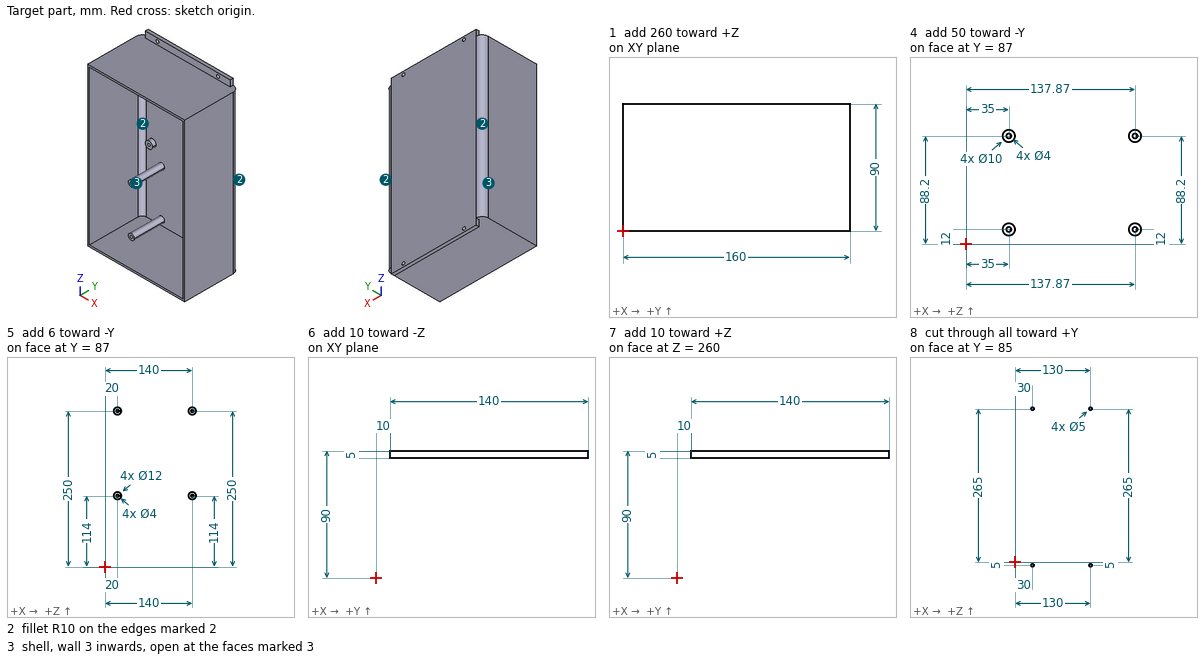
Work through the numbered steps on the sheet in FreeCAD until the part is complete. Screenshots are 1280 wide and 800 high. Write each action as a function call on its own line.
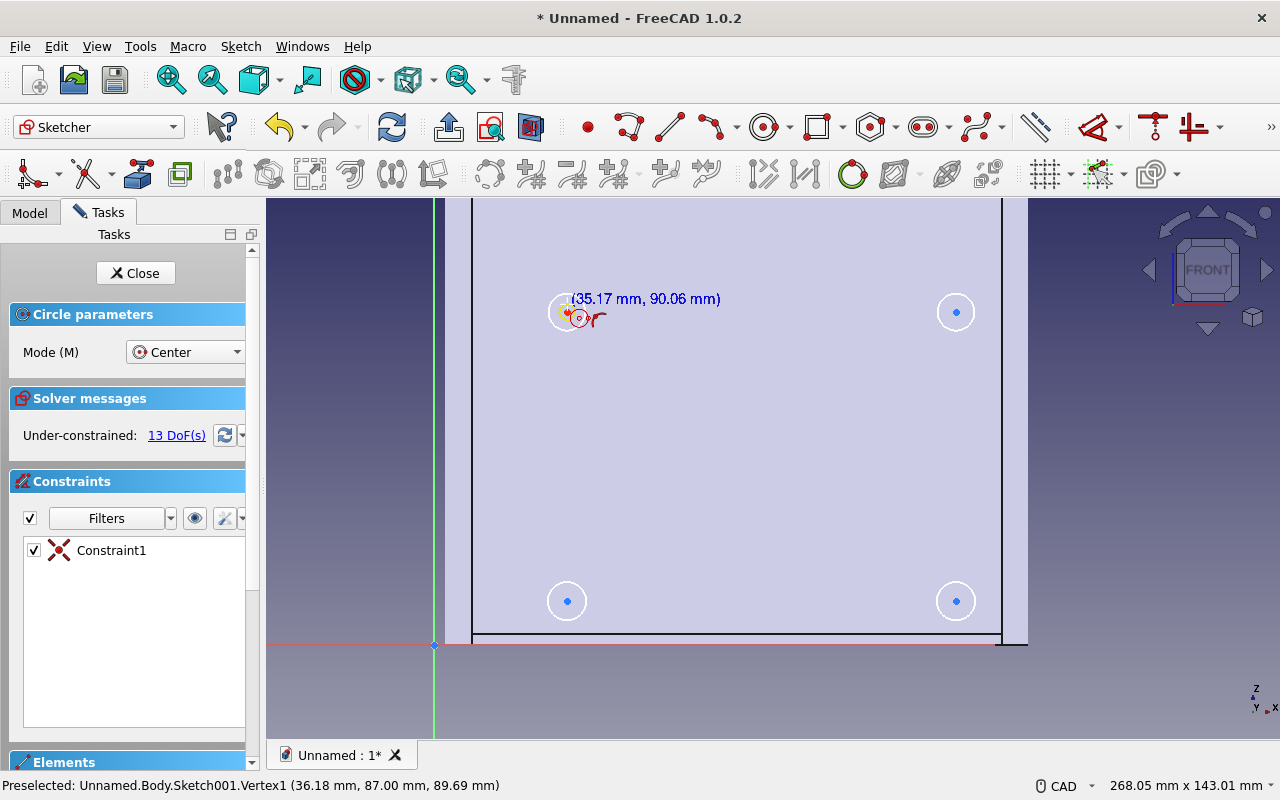
scroll(567, 600, up, 6)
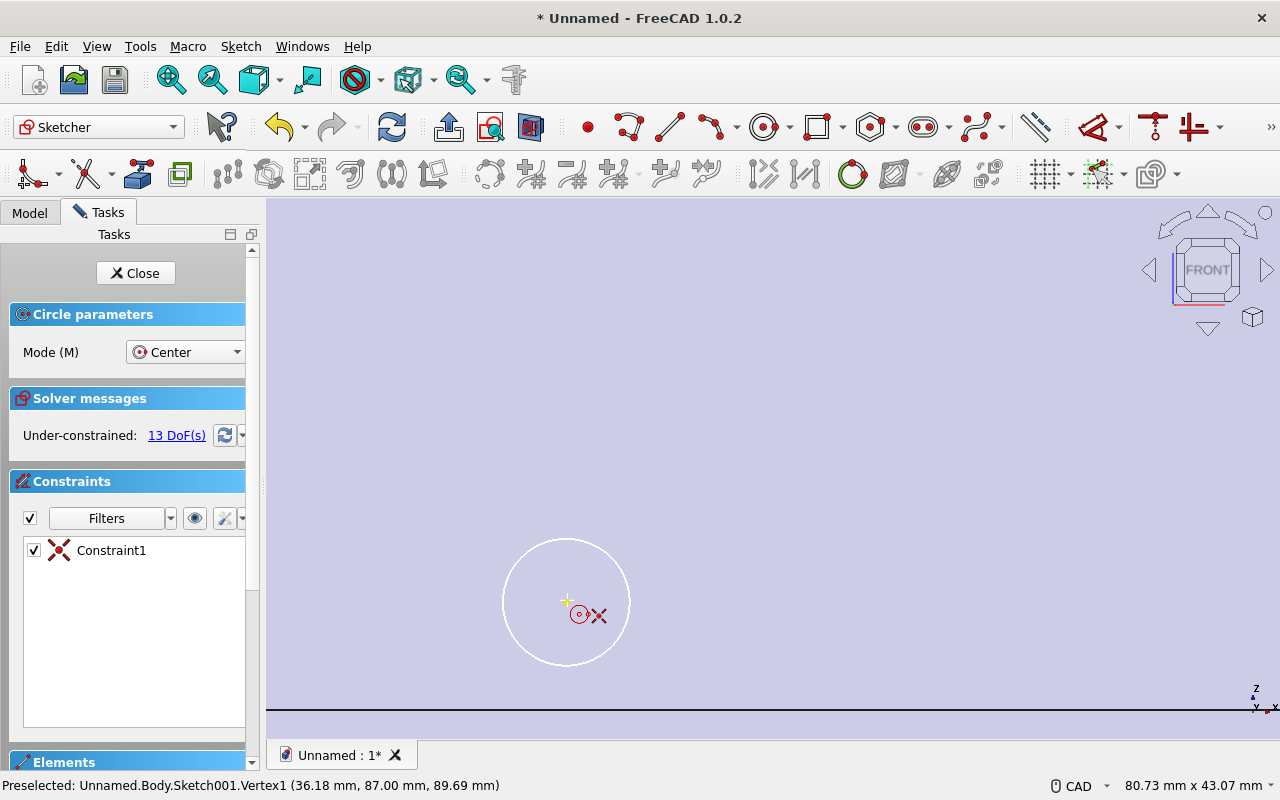
click(566, 602)
click(583, 580)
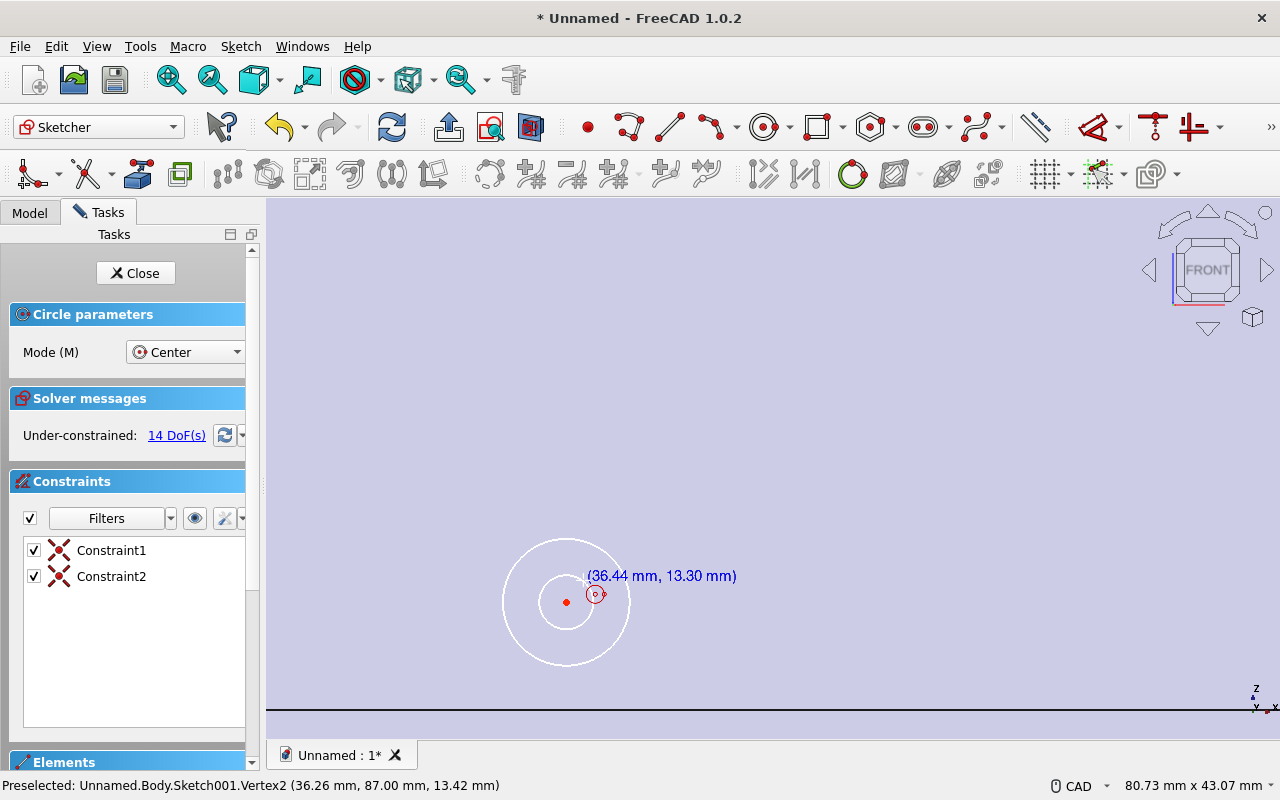
scroll(567, 600, down, 6)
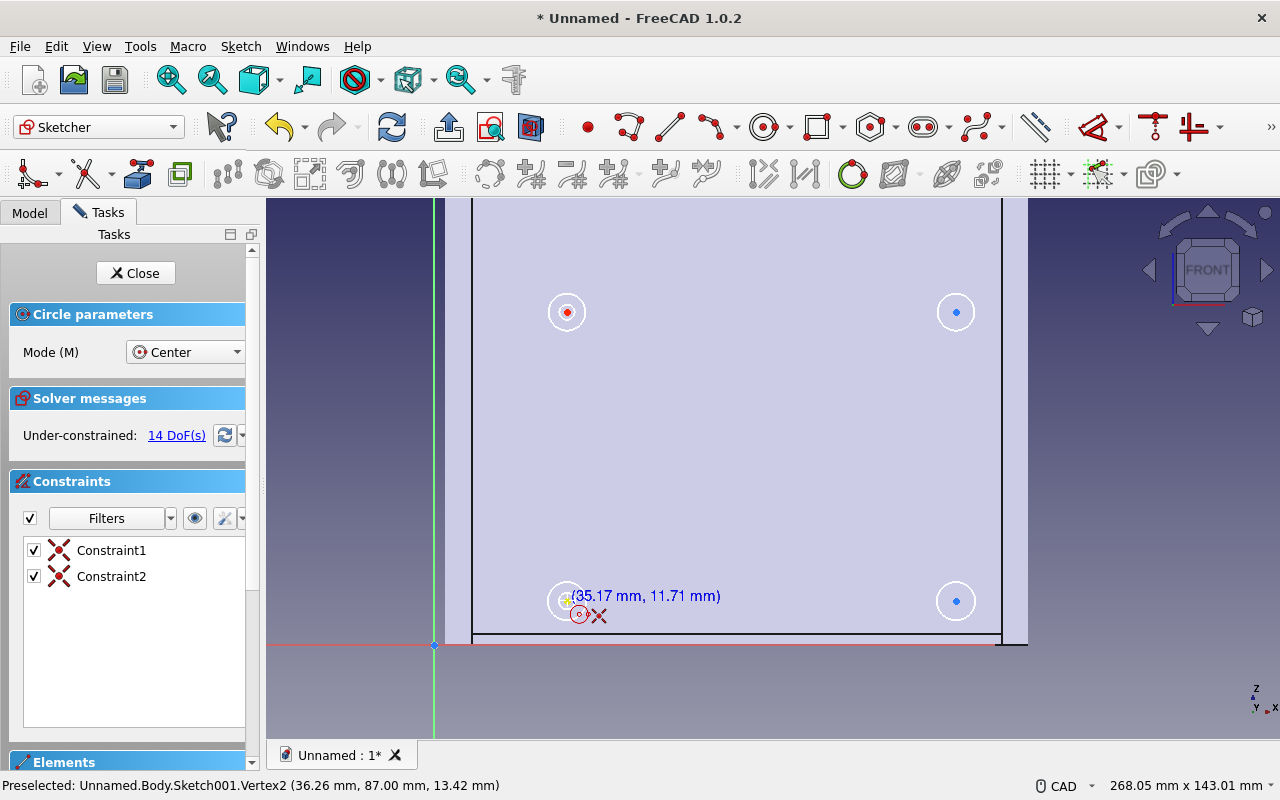
scroll(956, 600, up, 6)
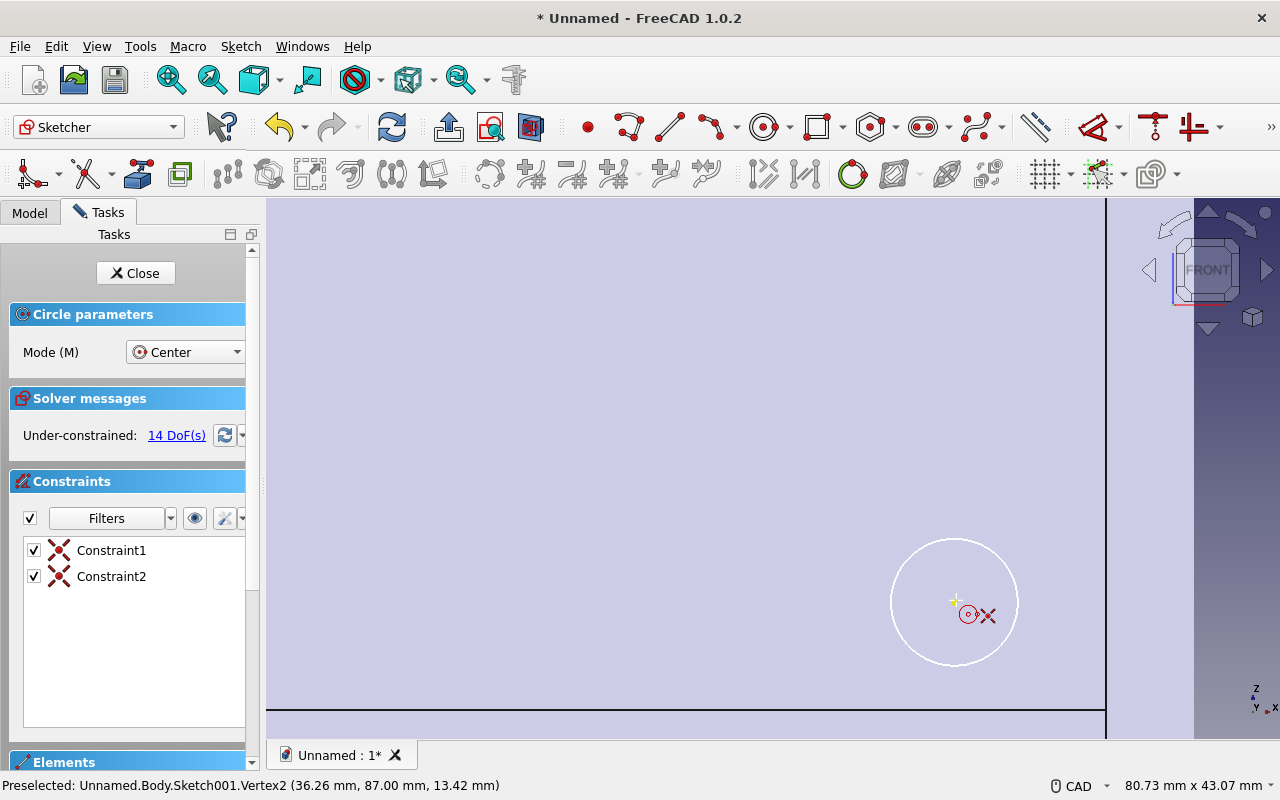
click(954, 602)
click(971, 580)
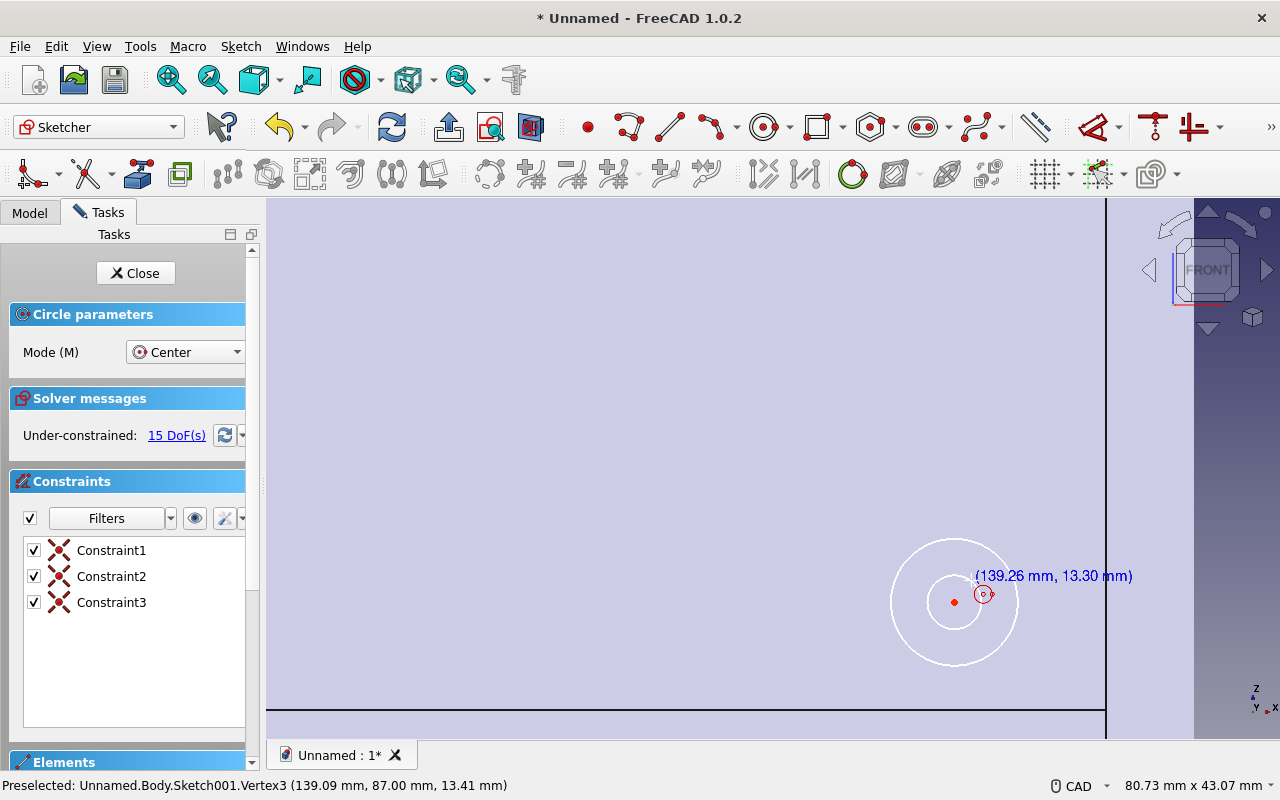
scroll(957, 600, down, 6)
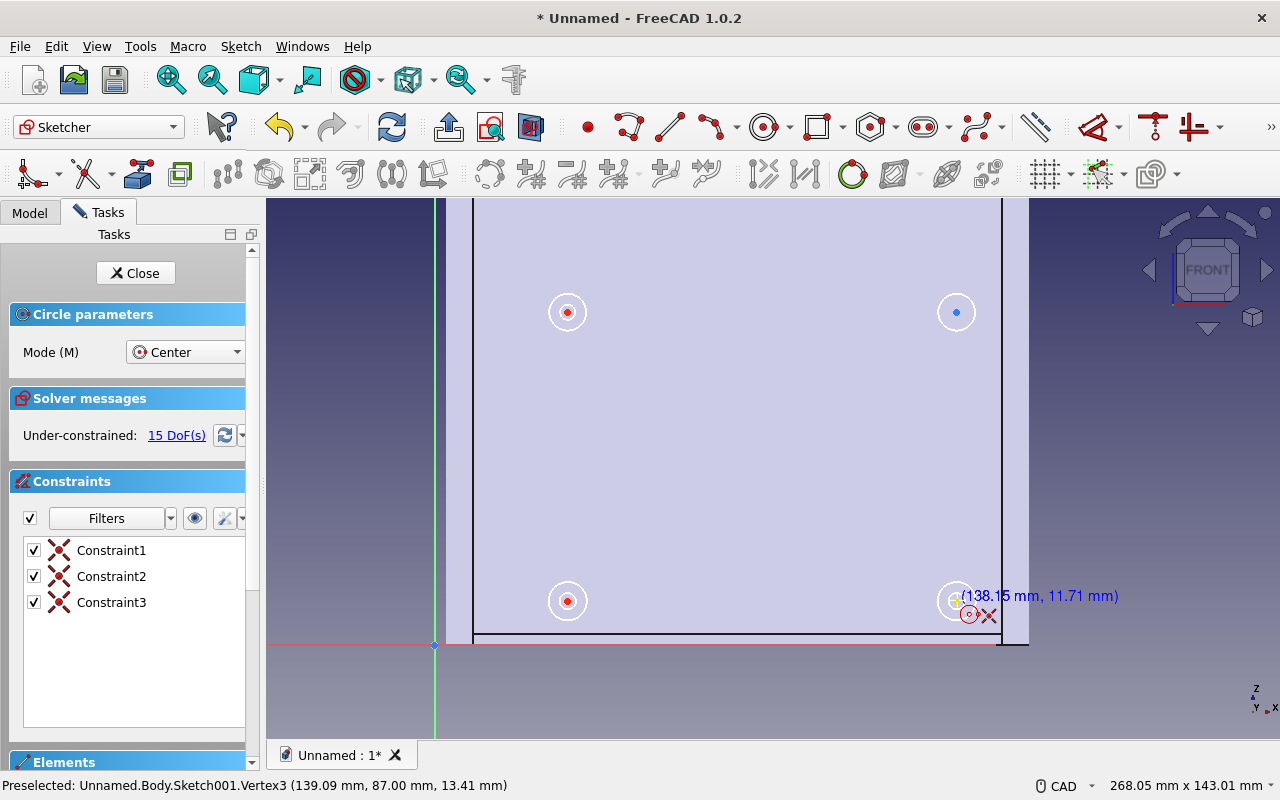
scroll(956, 311, up, 6)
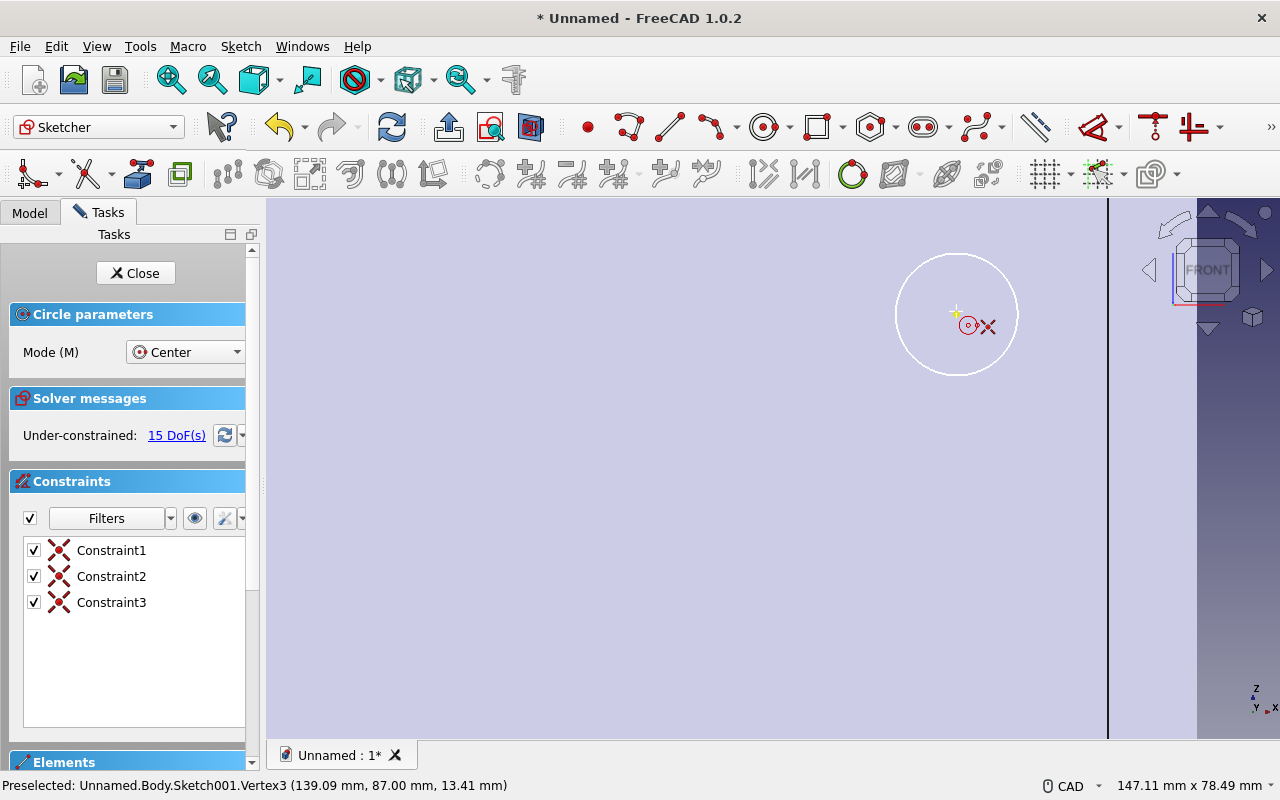
click(957, 314)
click(974, 294)
key(Escape)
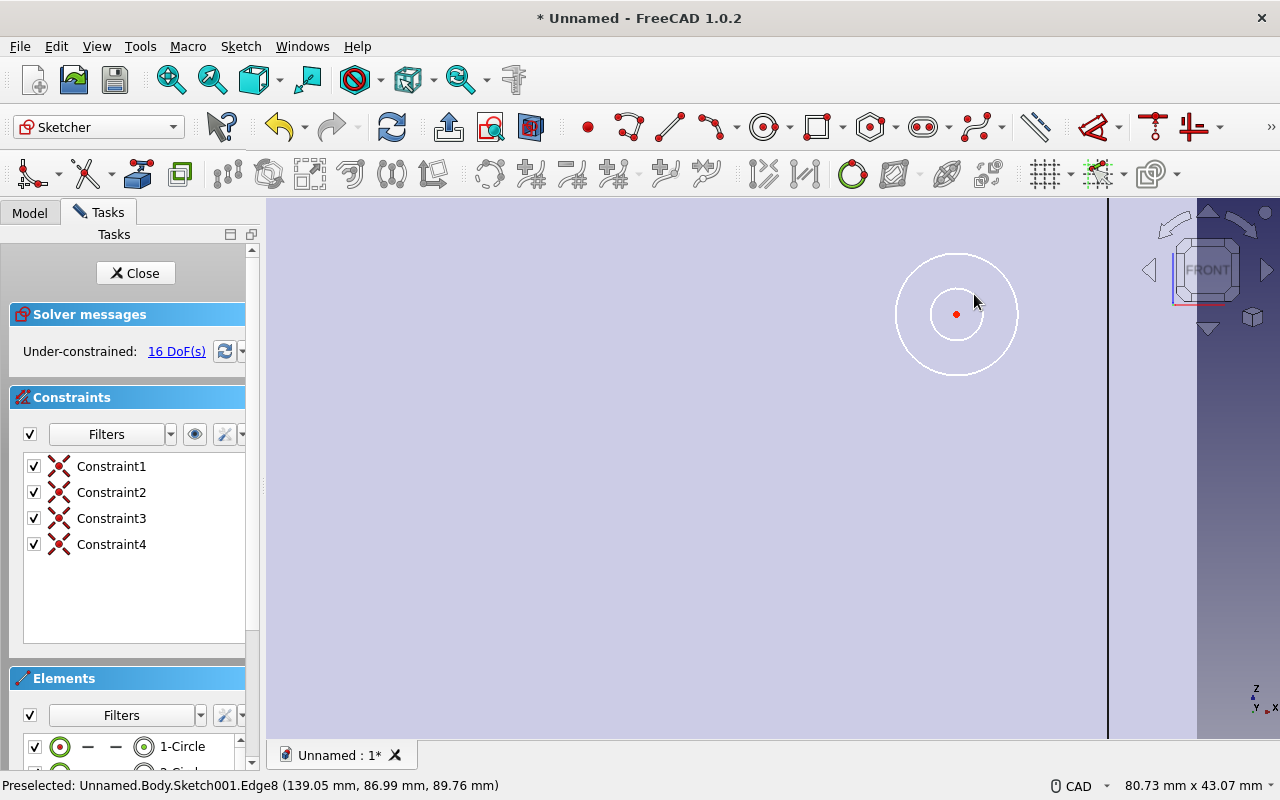
scroll(956, 311, down, 6)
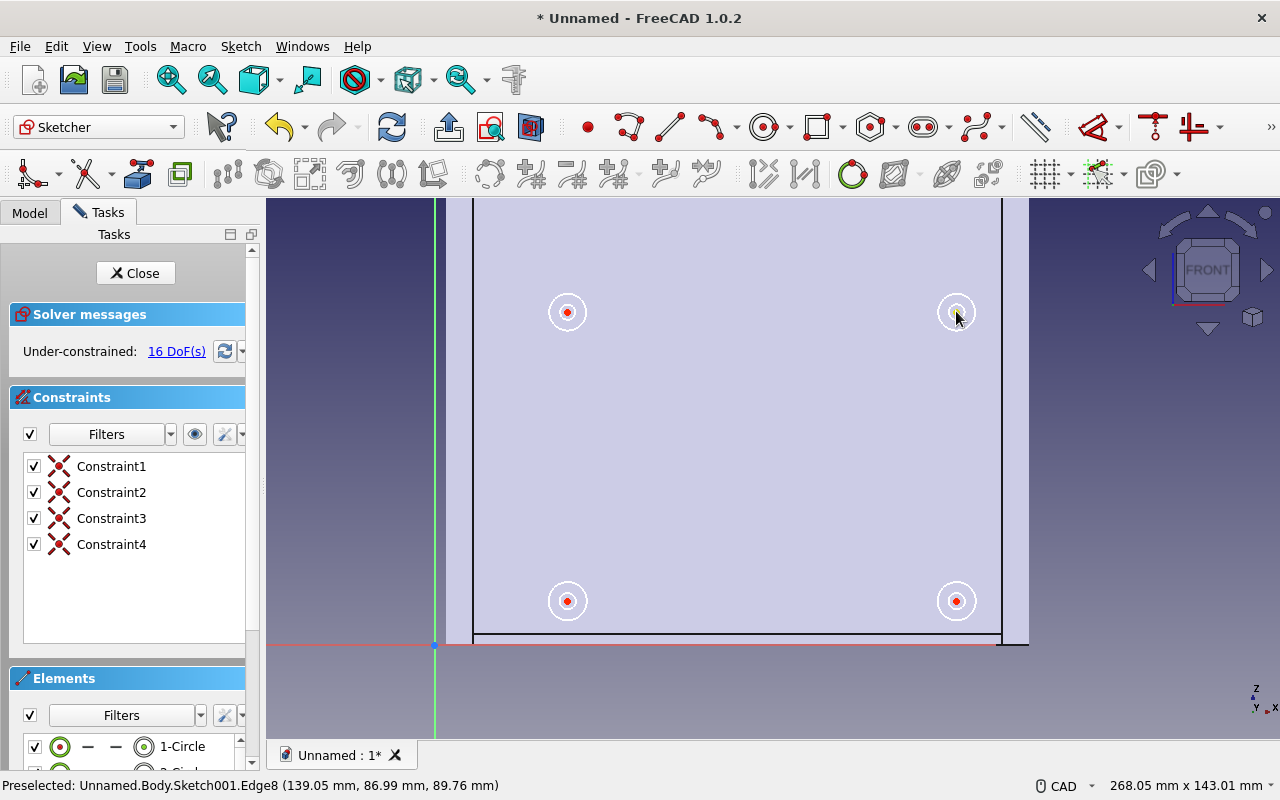
scroll(581, 299, up, 2)